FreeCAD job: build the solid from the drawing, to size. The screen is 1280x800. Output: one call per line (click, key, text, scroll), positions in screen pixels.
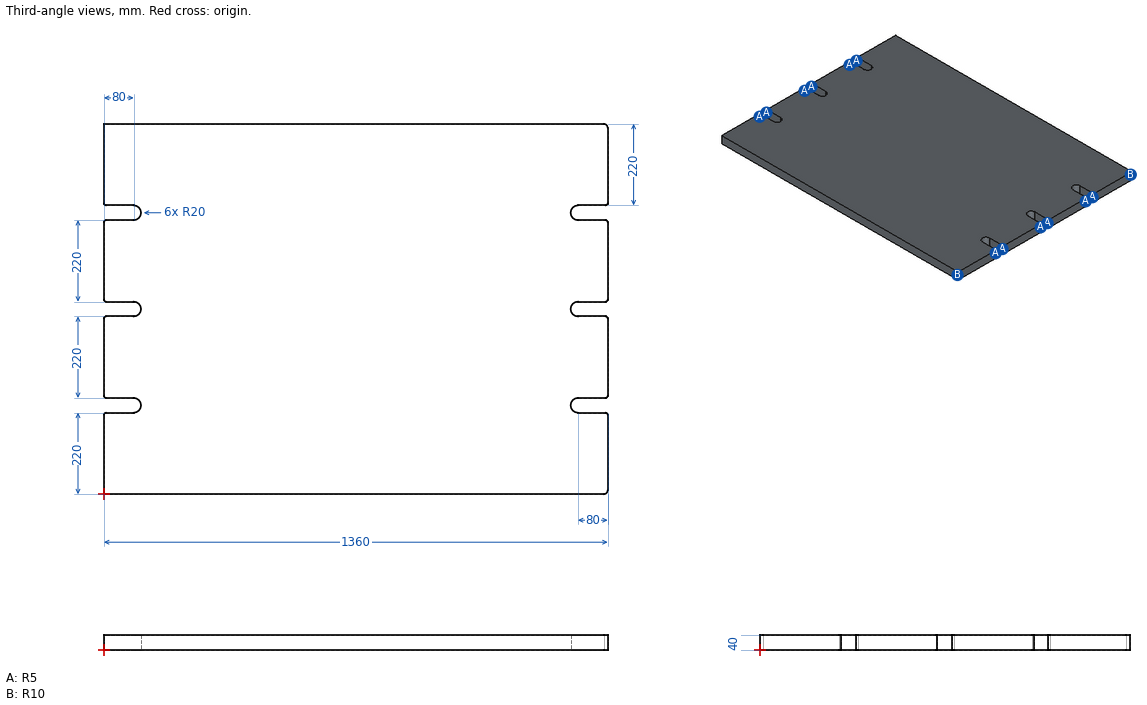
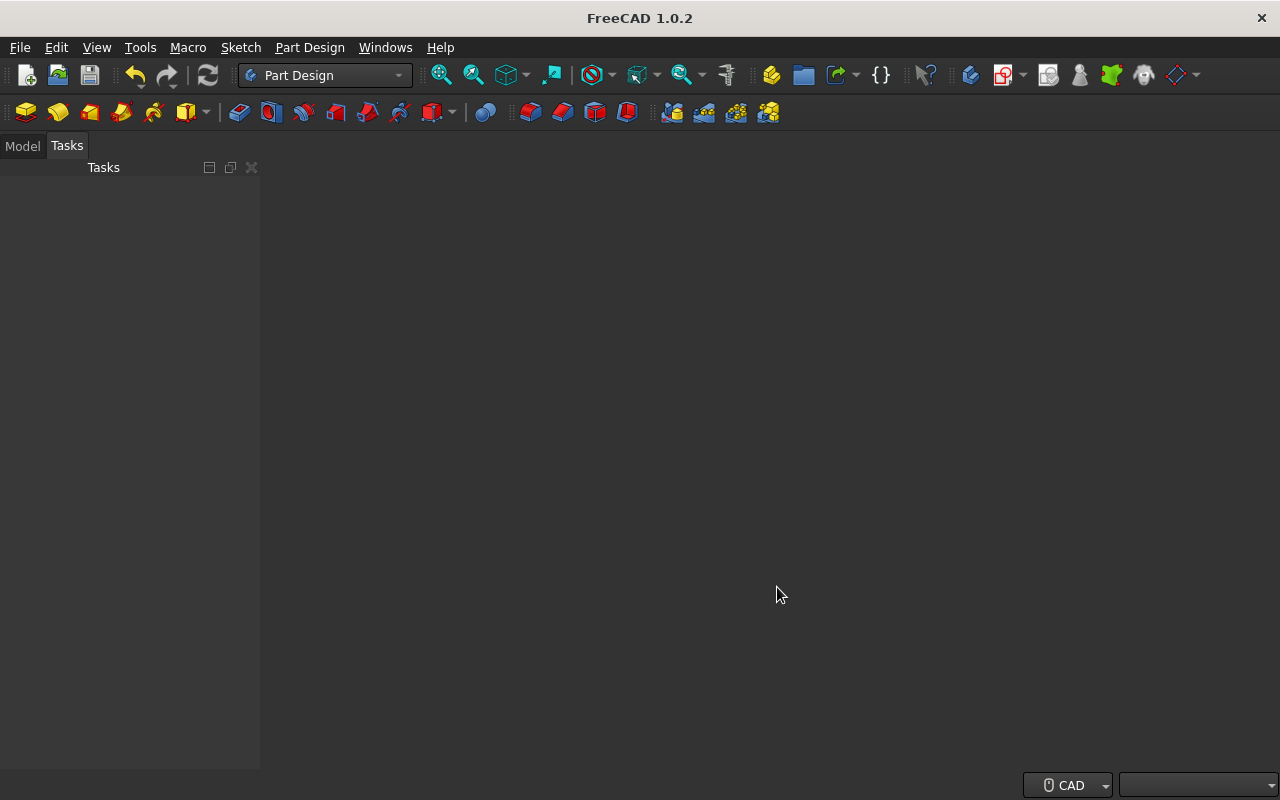
click(26, 76)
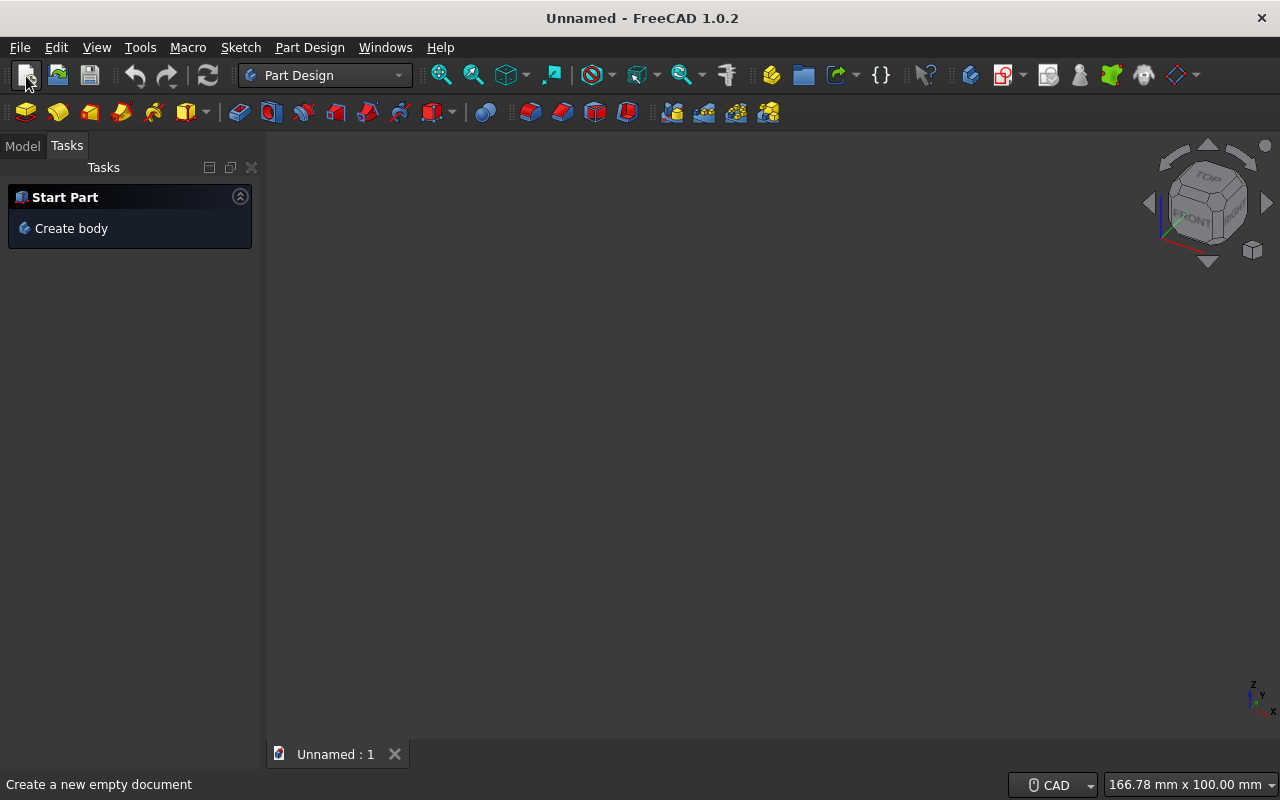
click(1004, 76)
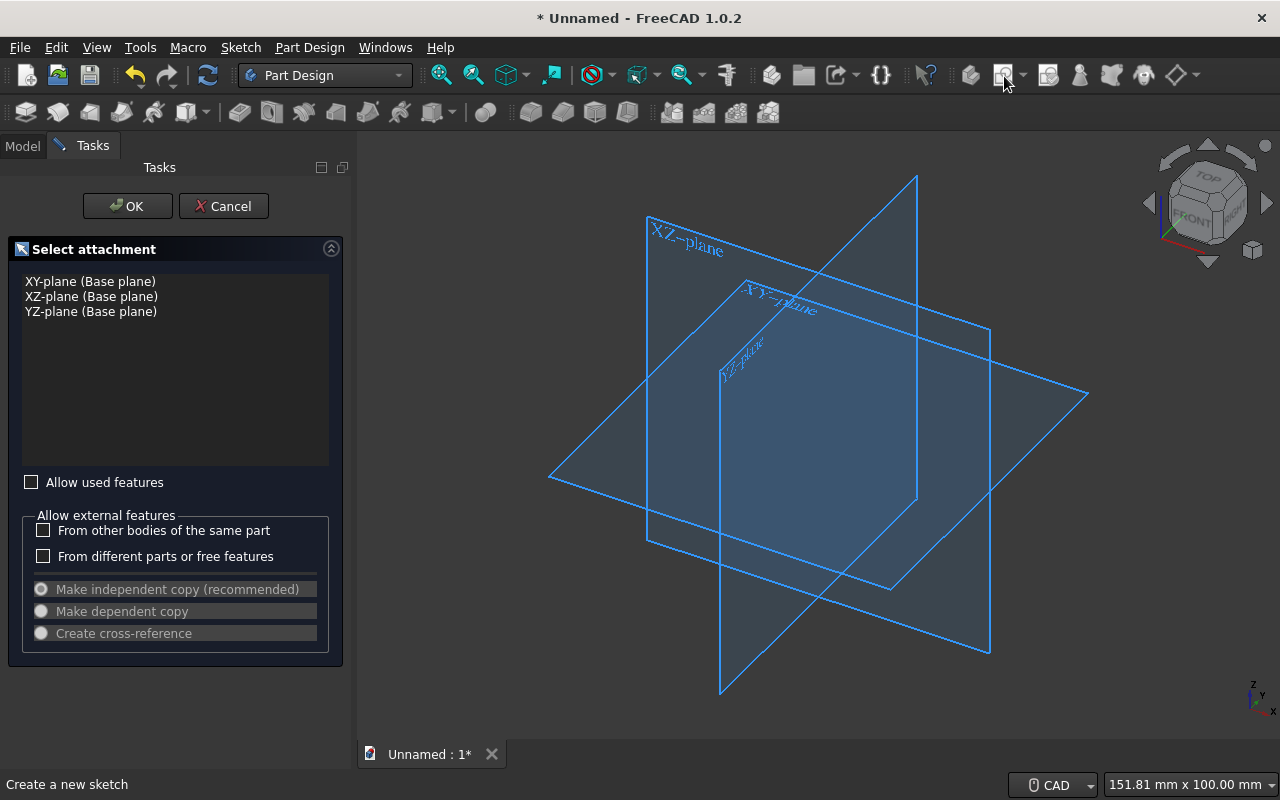
click(82, 282)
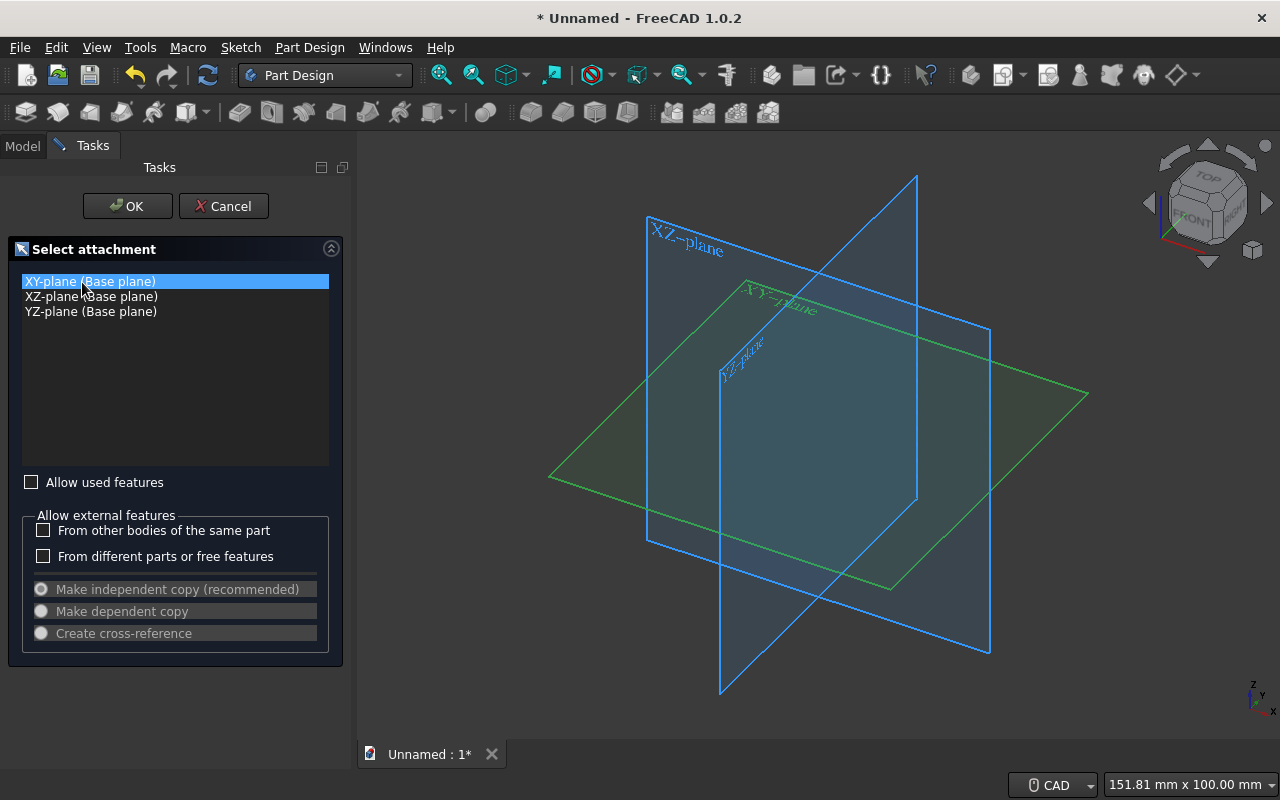
click(128, 206)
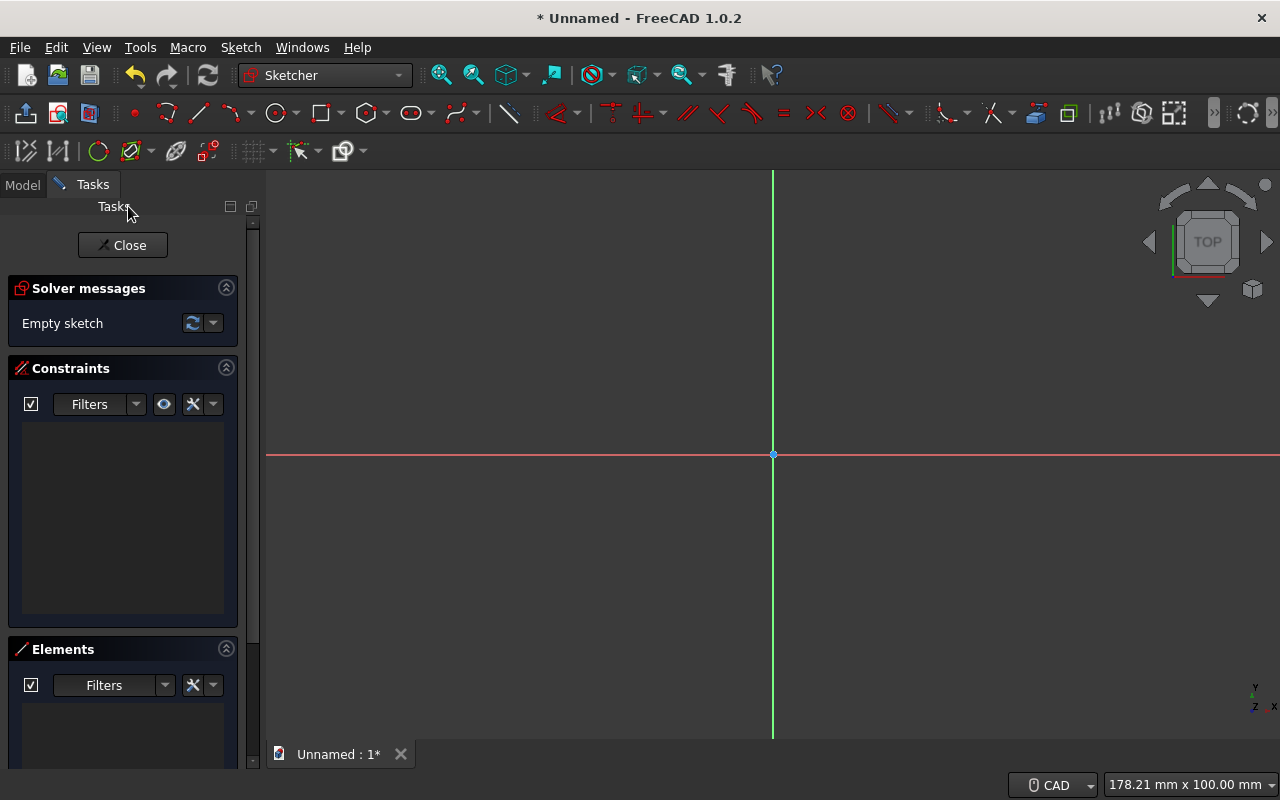
scroll(450, 639, down, 14)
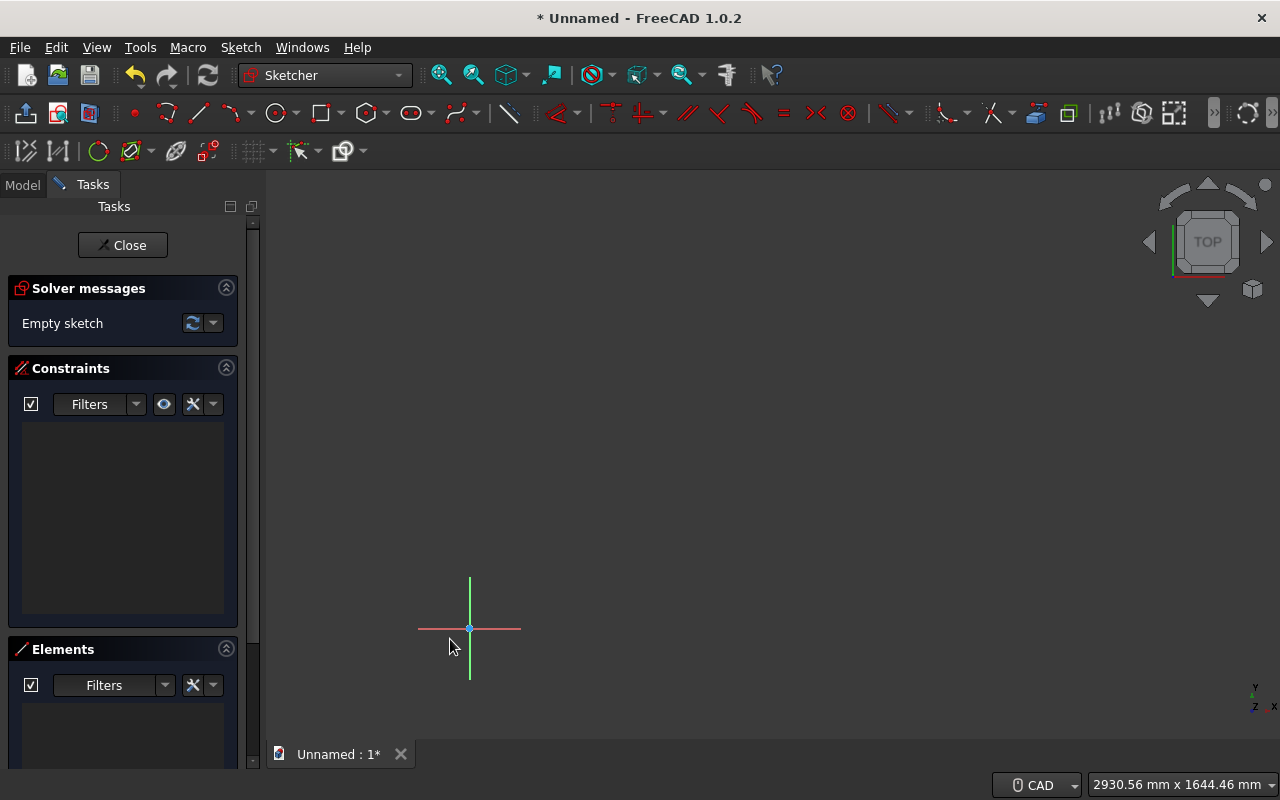
click(168, 114)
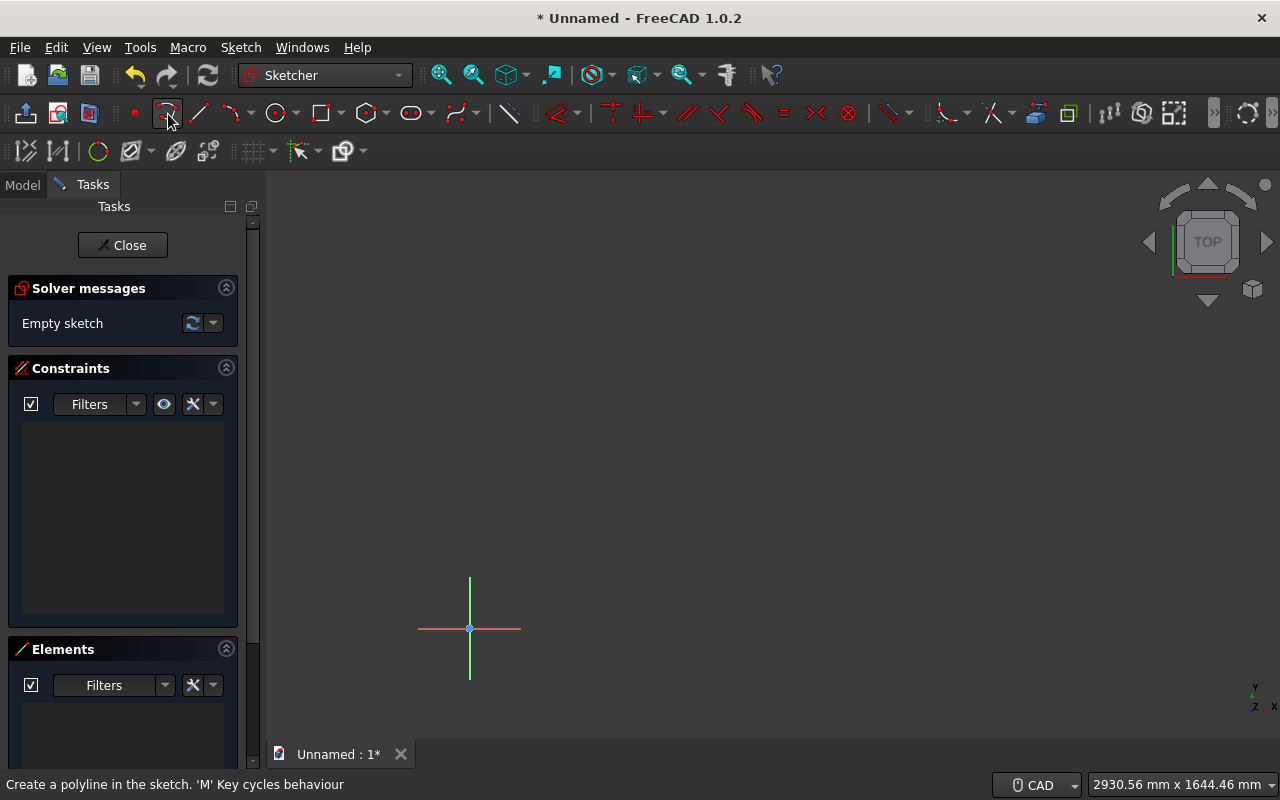
click(497, 373)
click(470, 373)
click(479, 449)
click(497, 449)
right_click(497, 449)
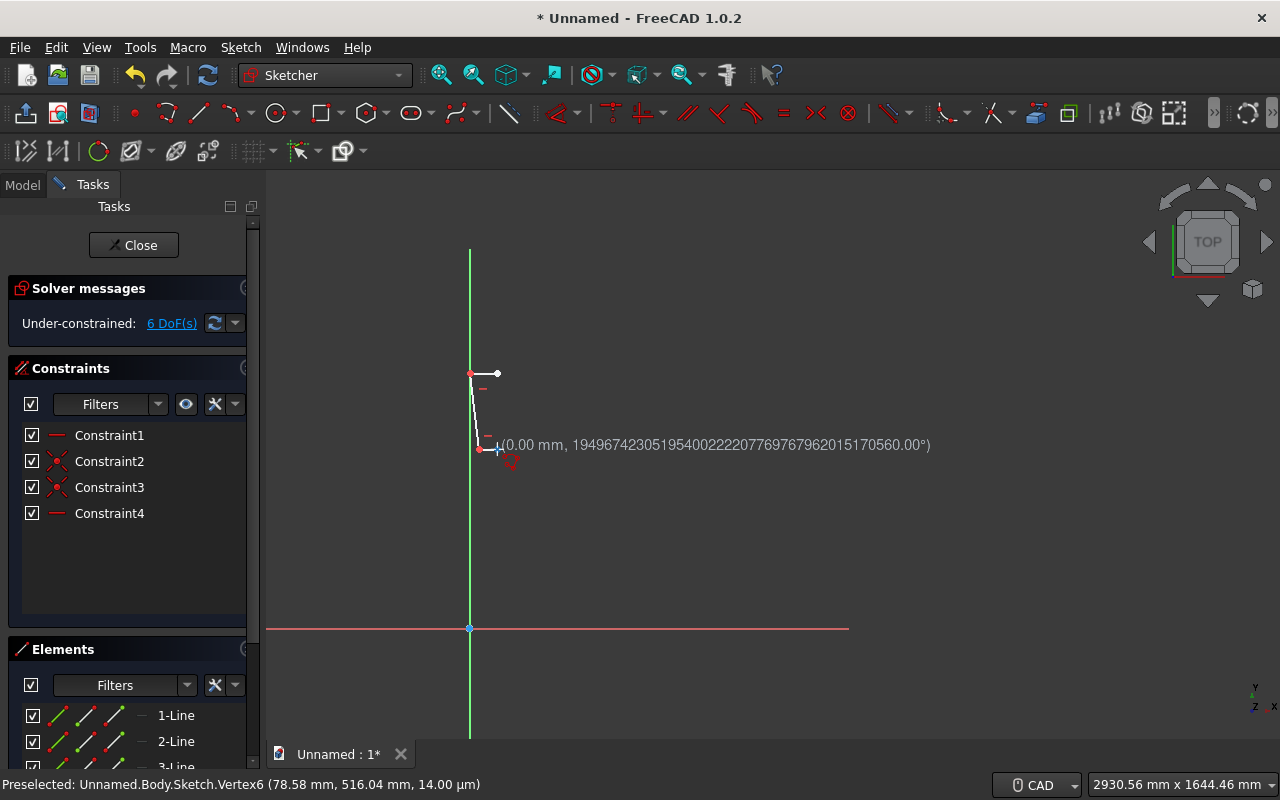
click(497, 462)
click(470, 462)
click(479, 539)
click(497, 539)
right_click(497, 539)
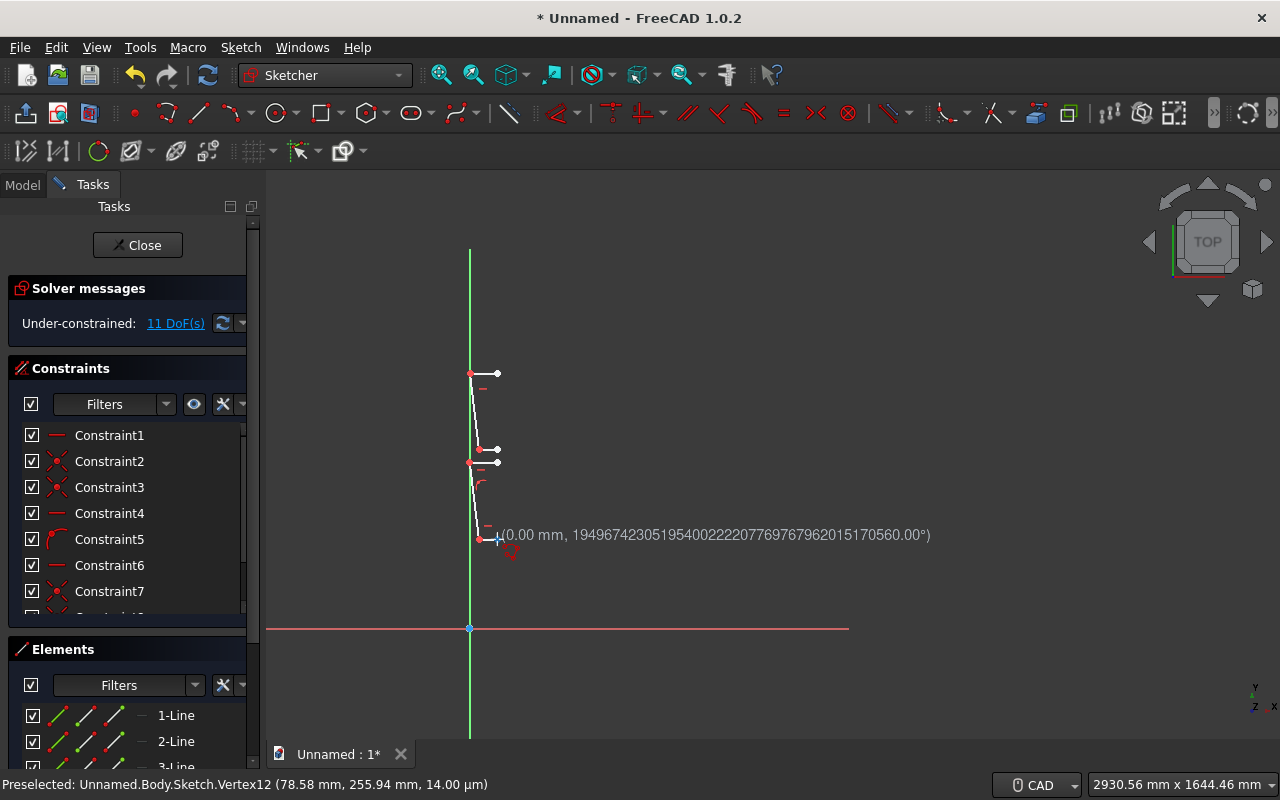
click(497, 552)
click(470, 552)
click(470, 629)
click(940, 620)
click(940, 552)
click(913, 552)
right_click(913, 552)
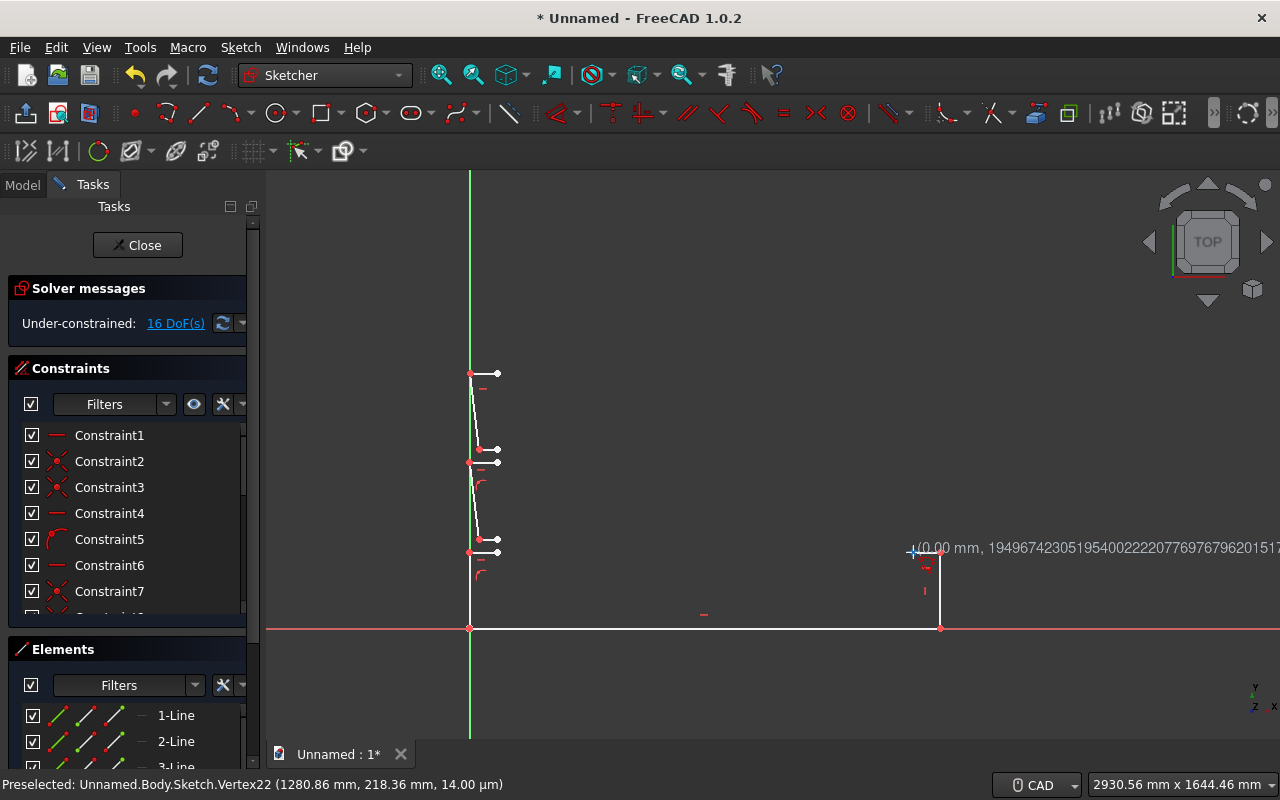
click(913, 539)
click(940, 539)
click(940, 462)
click(913, 462)
right_click(913, 462)